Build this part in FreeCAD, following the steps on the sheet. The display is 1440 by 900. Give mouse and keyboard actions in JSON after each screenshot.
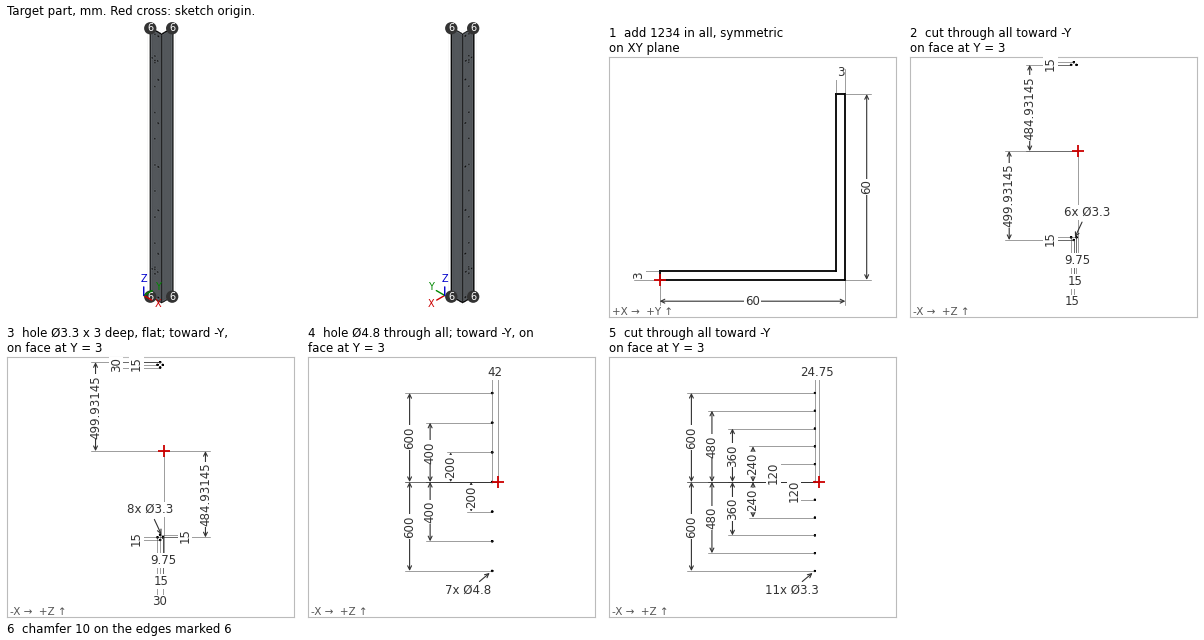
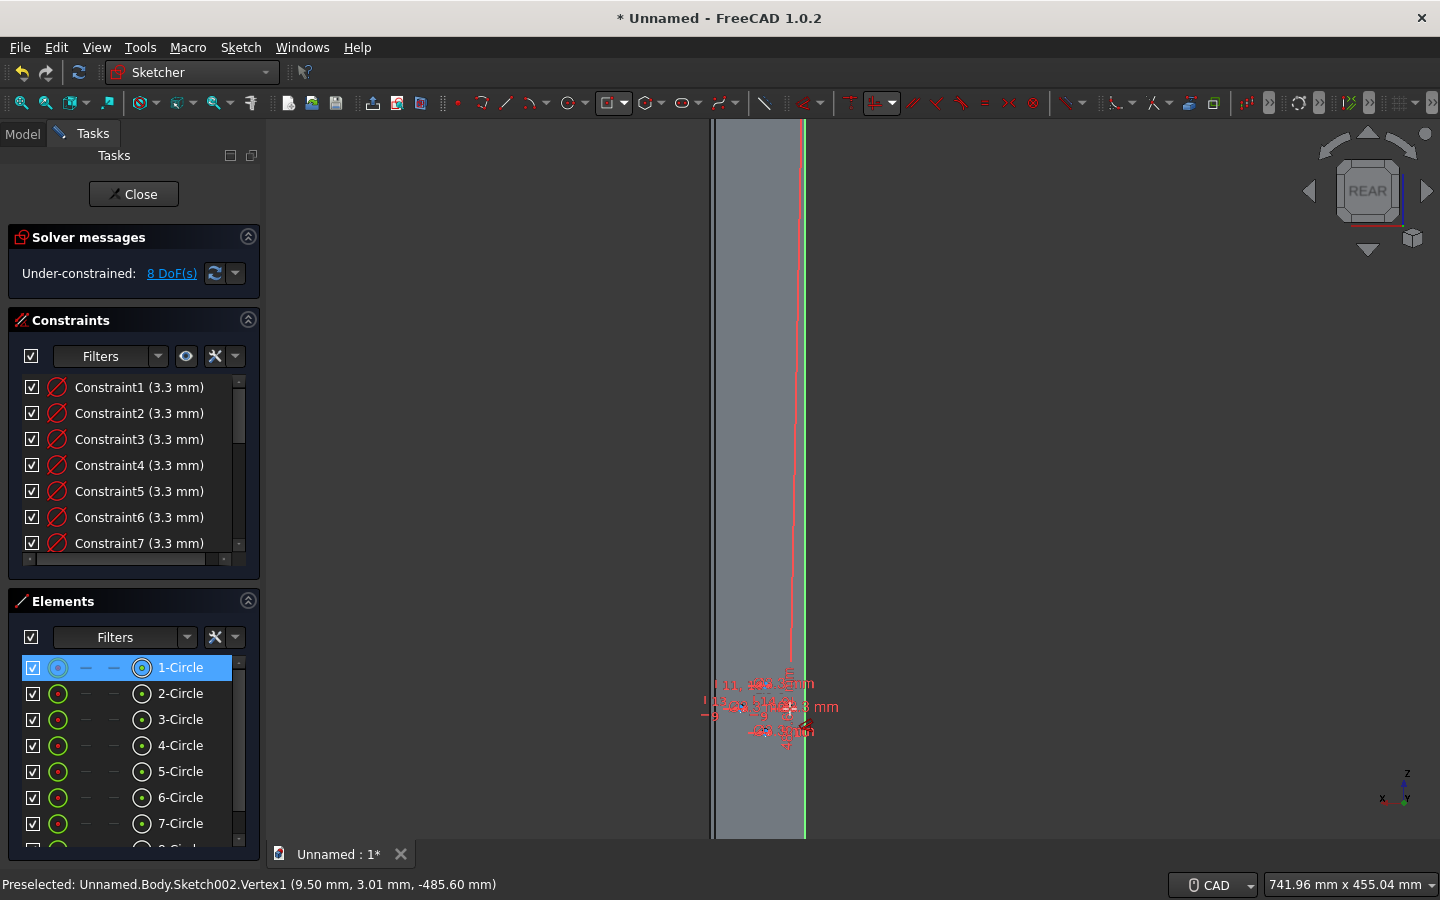
{"action": "left_click", "coordinate": [741, 709]}
{"action": "left_click", "coordinate": [748, 743]}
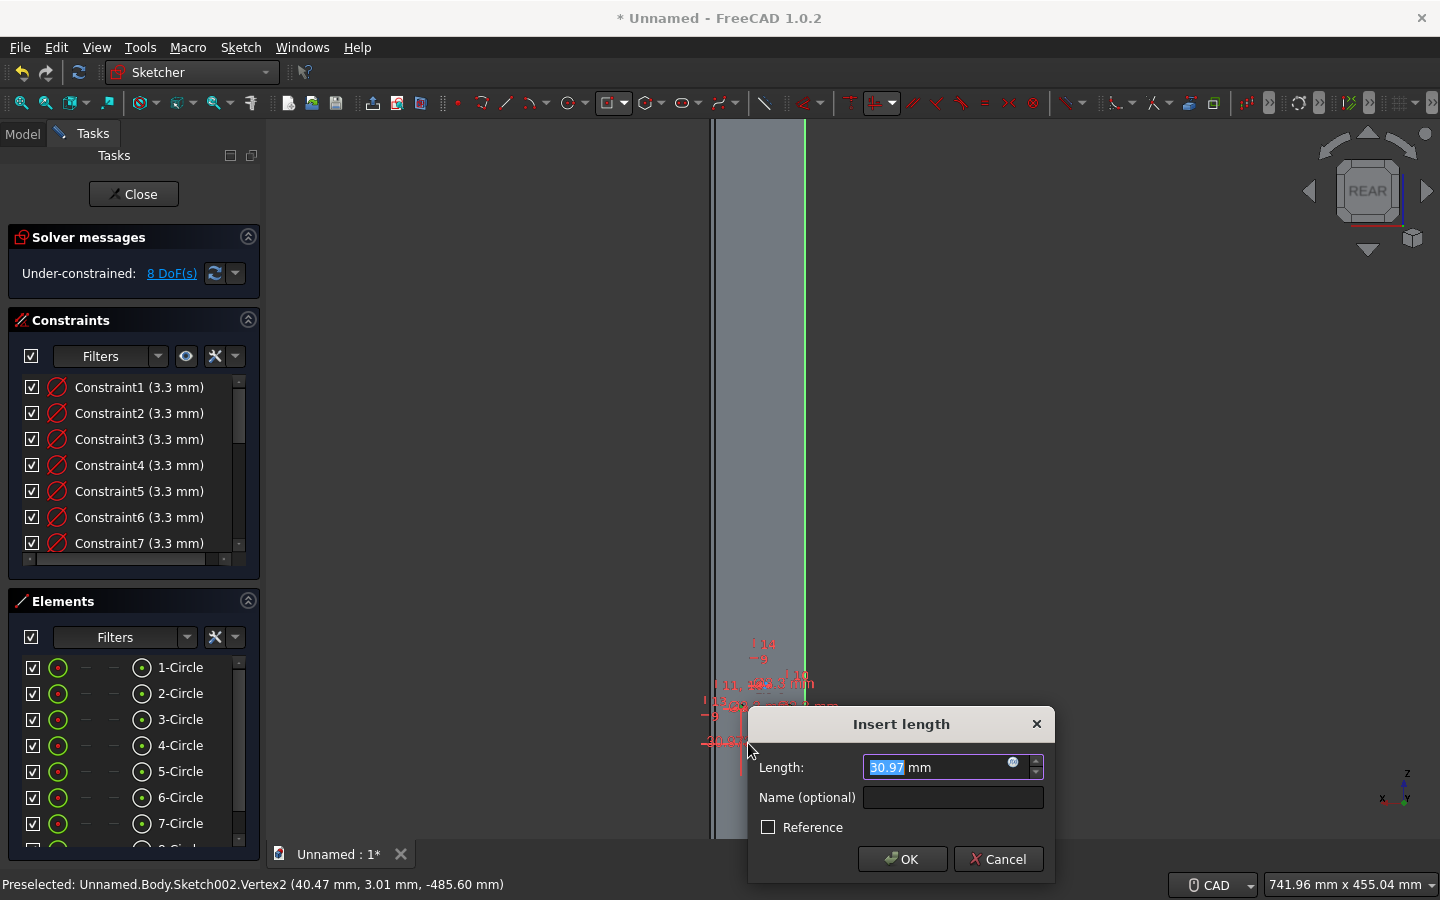
{"action": "type", "text": "30"}
{"action": "key", "text": "Return"}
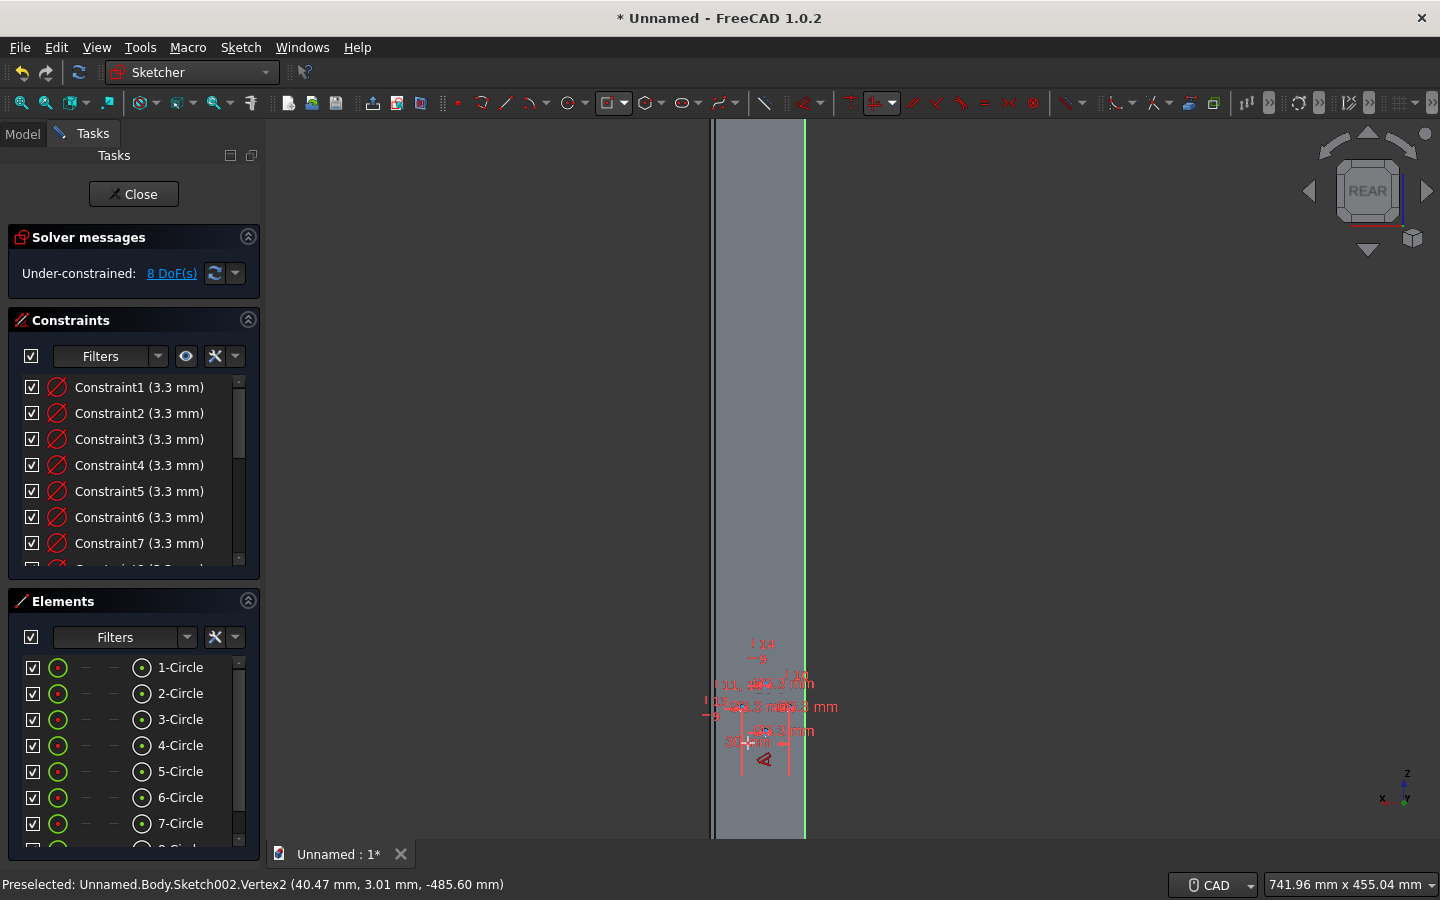
{"action": "scroll", "coordinate": [789, 709], "scroll_direction": "up", "scroll_amount": 3}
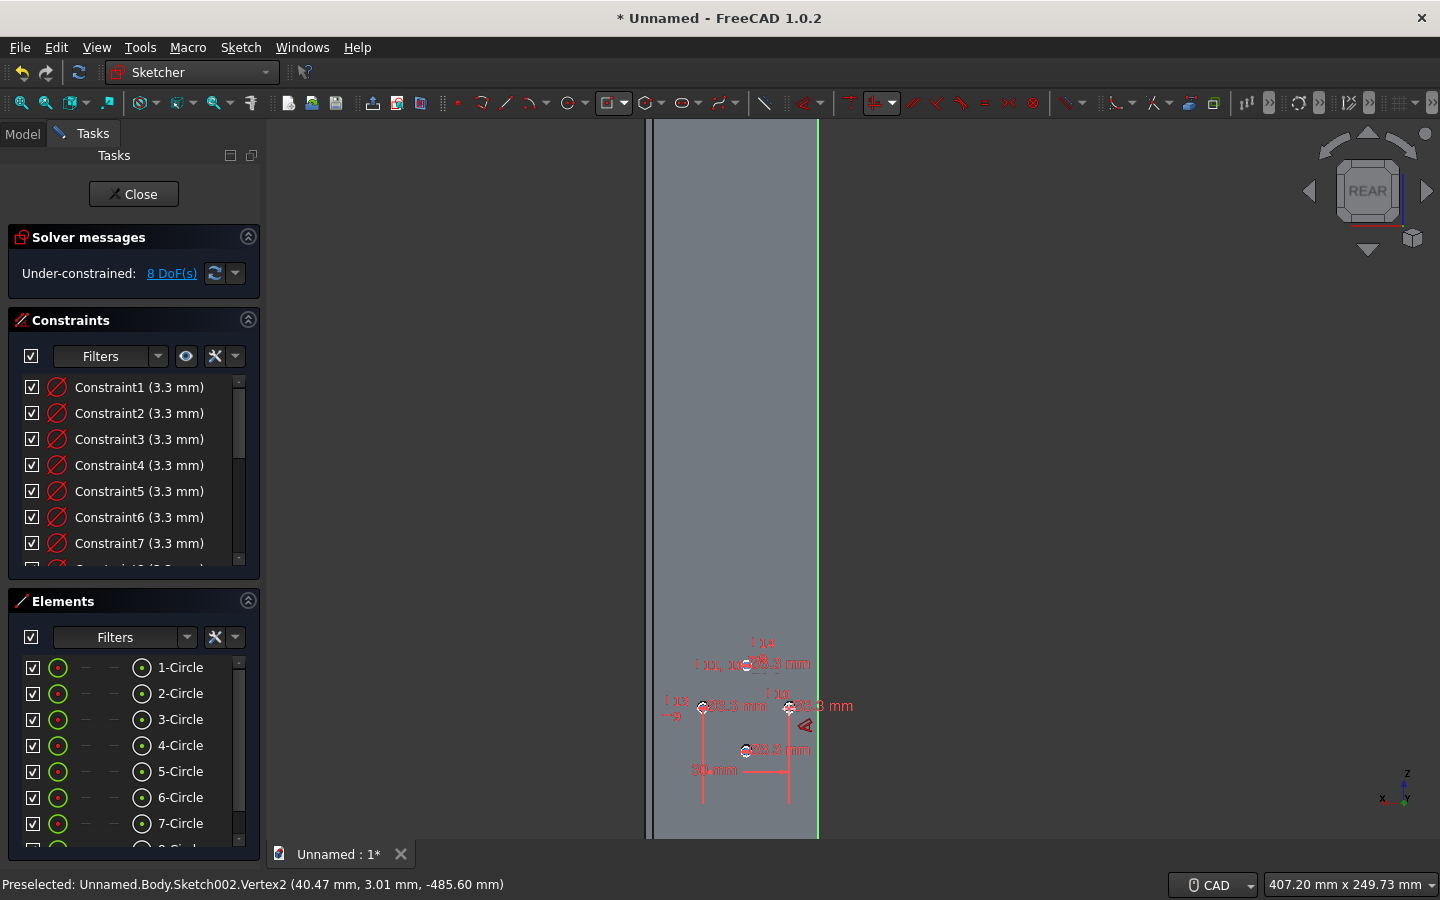
{"action": "left_click", "coordinate": [789, 708]}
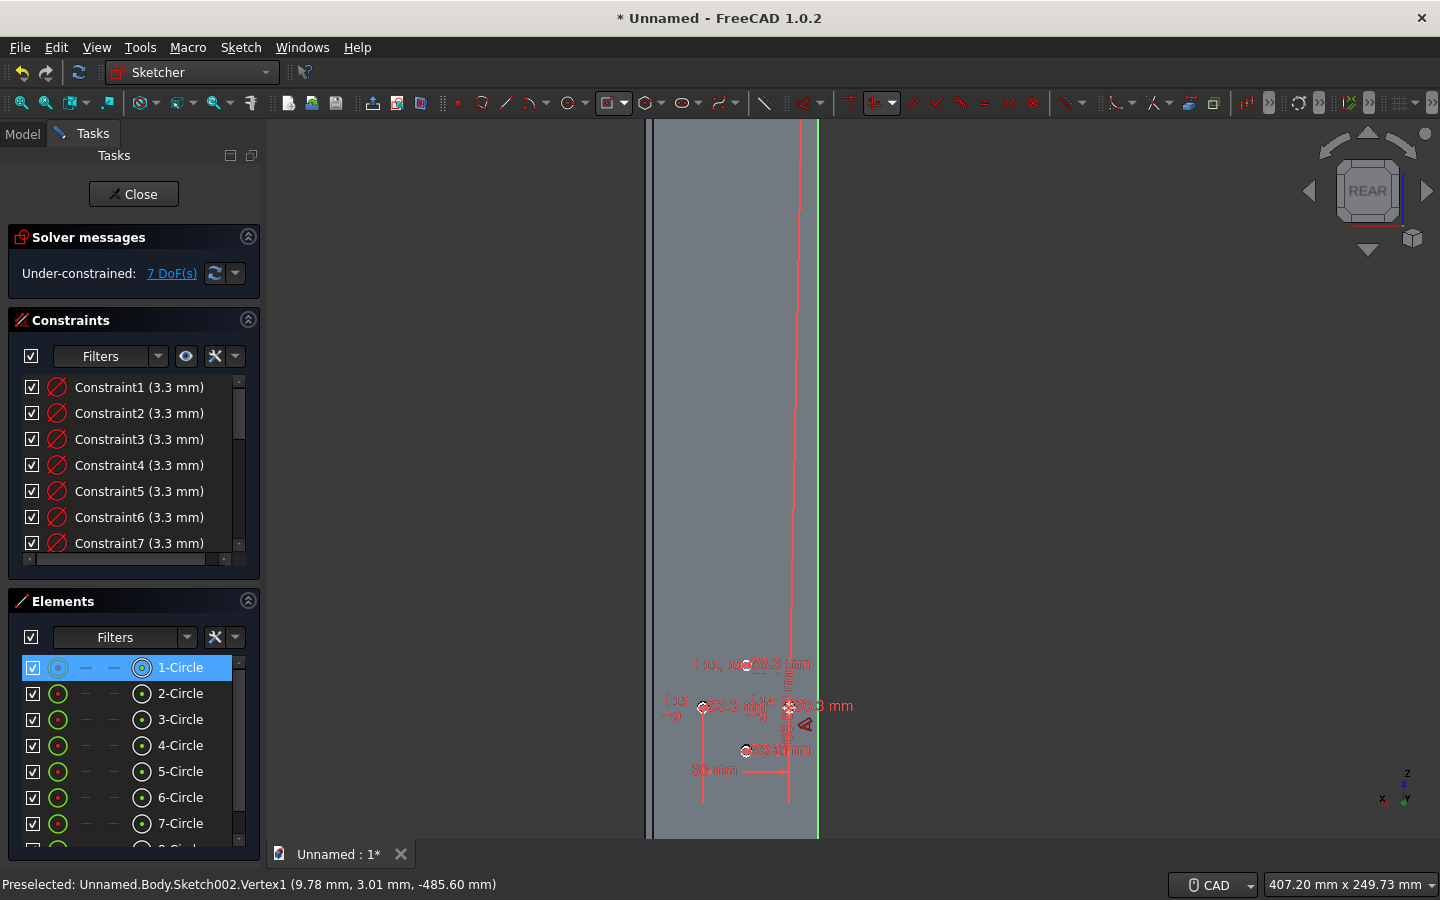
{"action": "left_click", "coordinate": [746, 666]}
{"action": "left_click", "coordinate": [768, 742]}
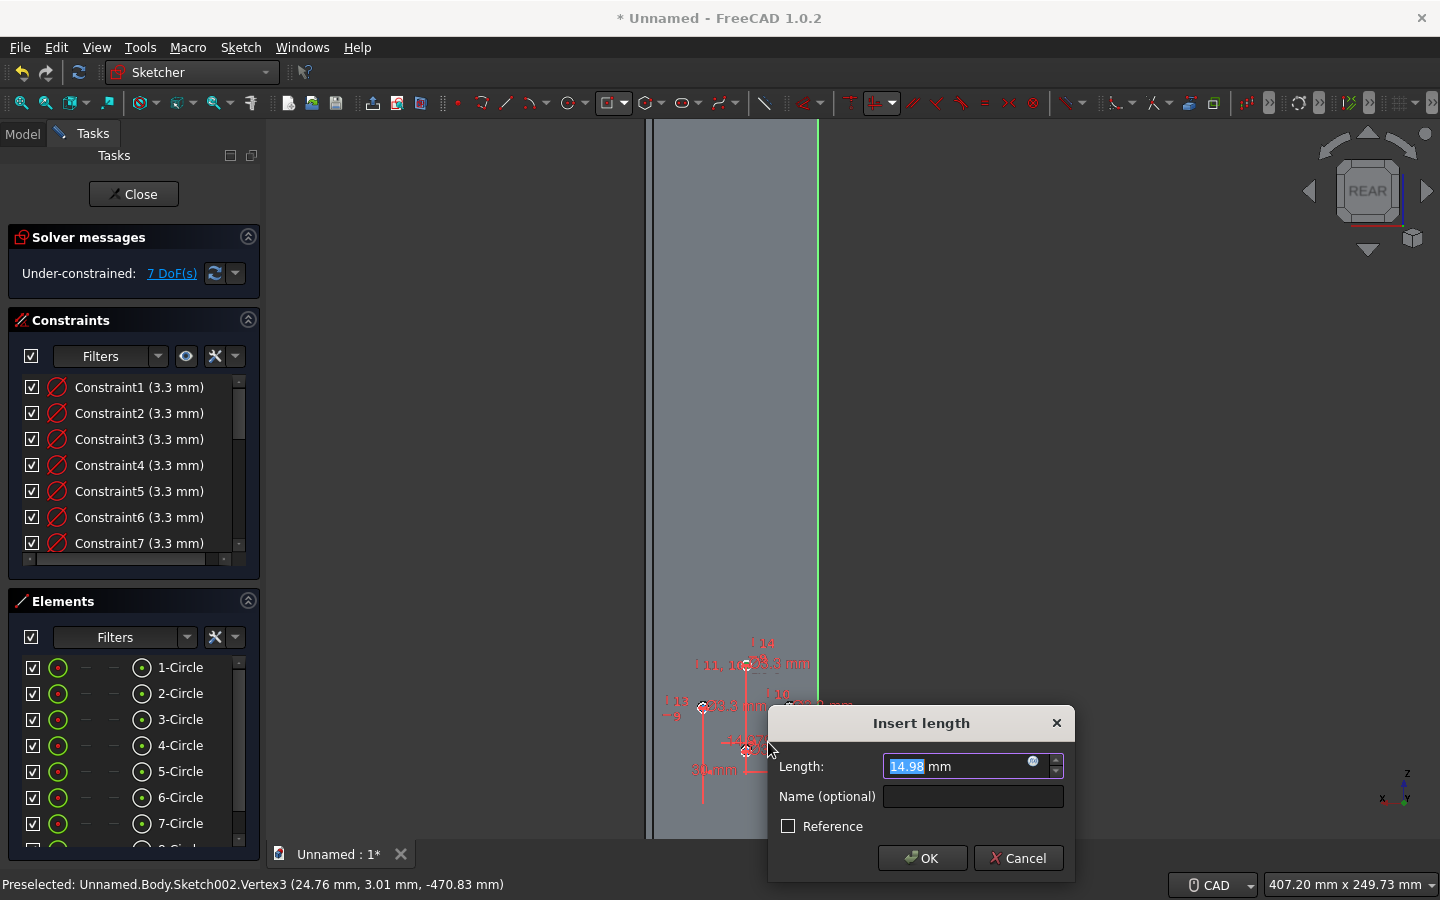
{"action": "type", "text": "15"}
{"action": "key", "text": "Return"}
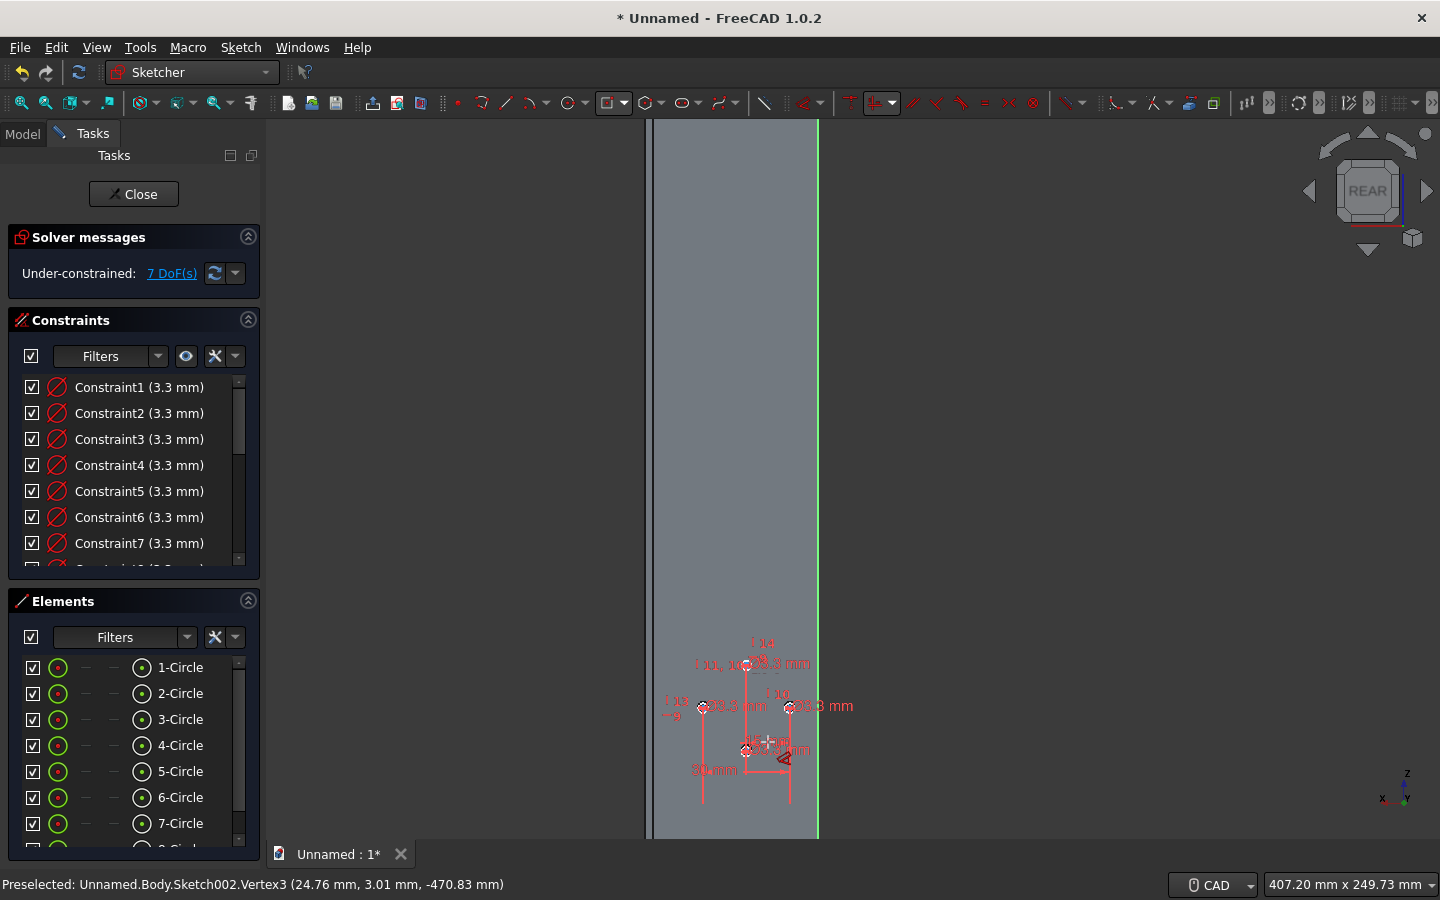
{"action": "left_click", "coordinate": [790, 708]}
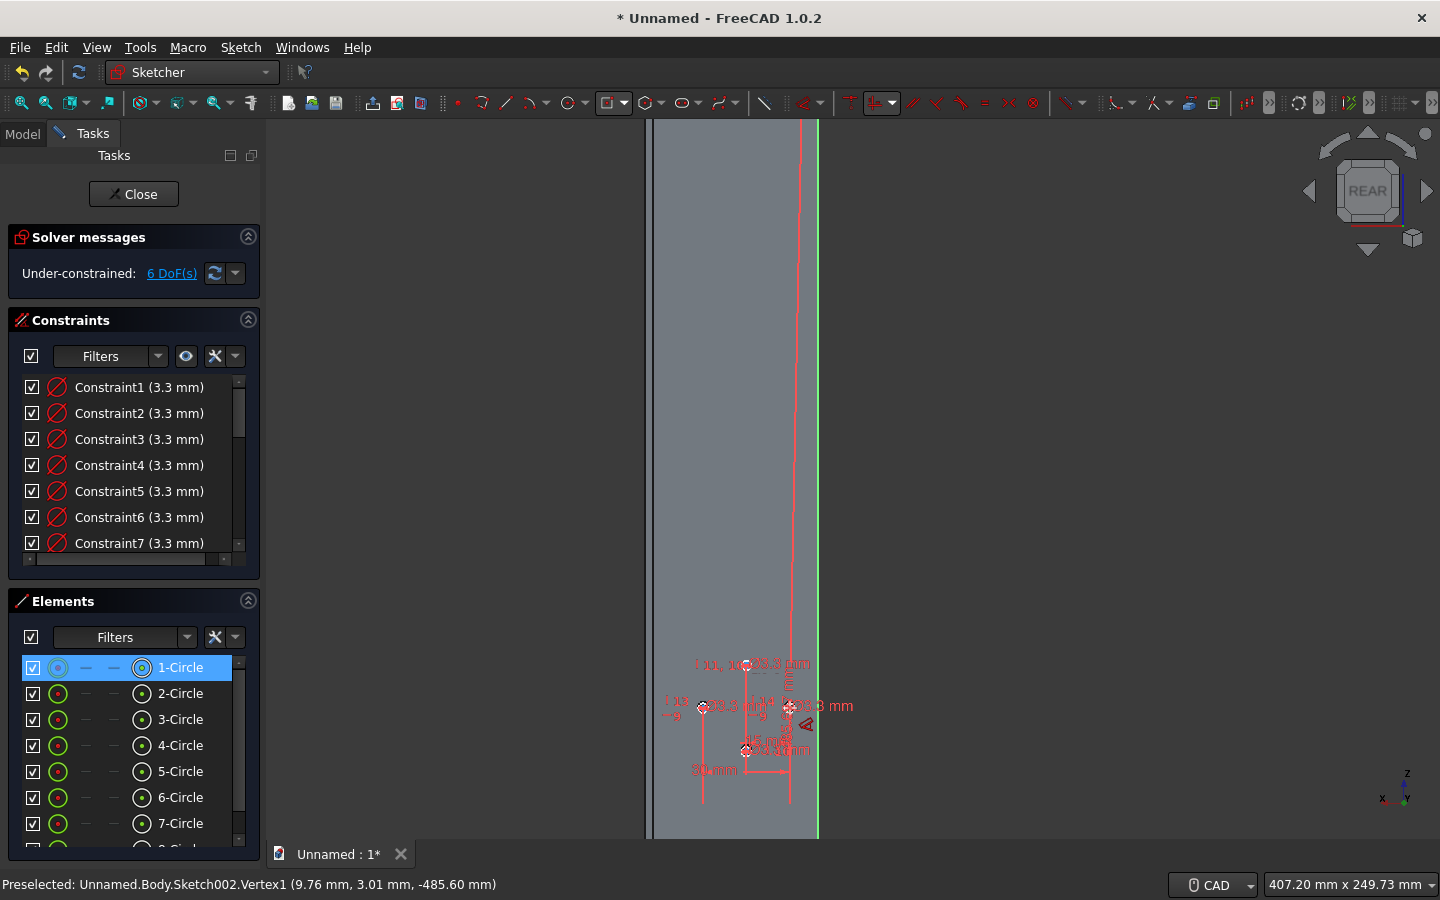
{"action": "left_click", "coordinate": [746, 666]}
{"action": "left_click", "coordinate": [712, 687]}